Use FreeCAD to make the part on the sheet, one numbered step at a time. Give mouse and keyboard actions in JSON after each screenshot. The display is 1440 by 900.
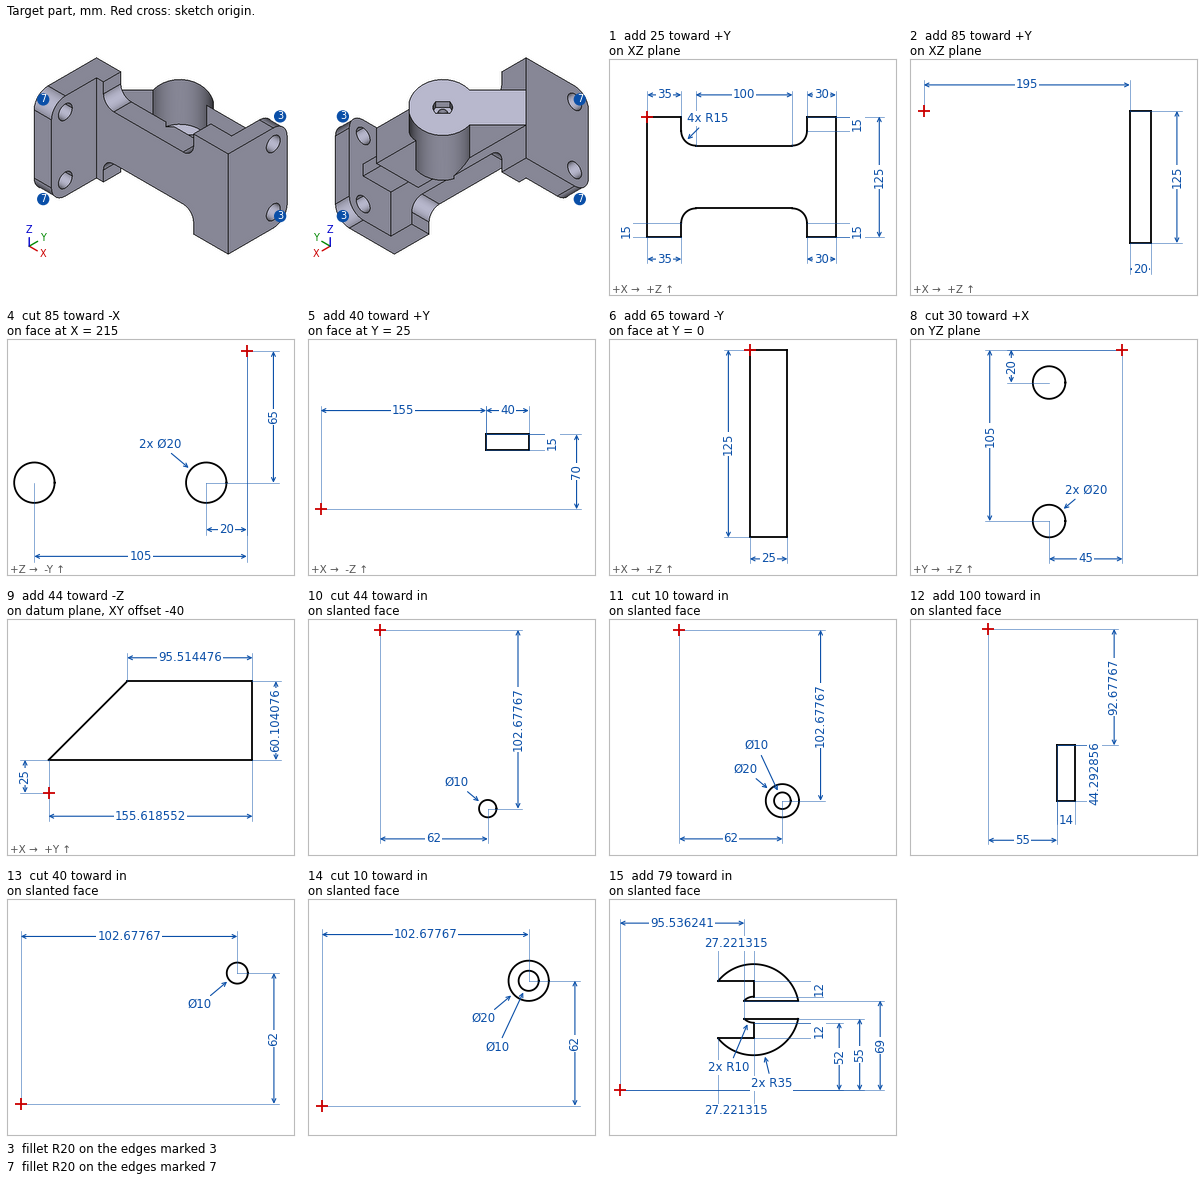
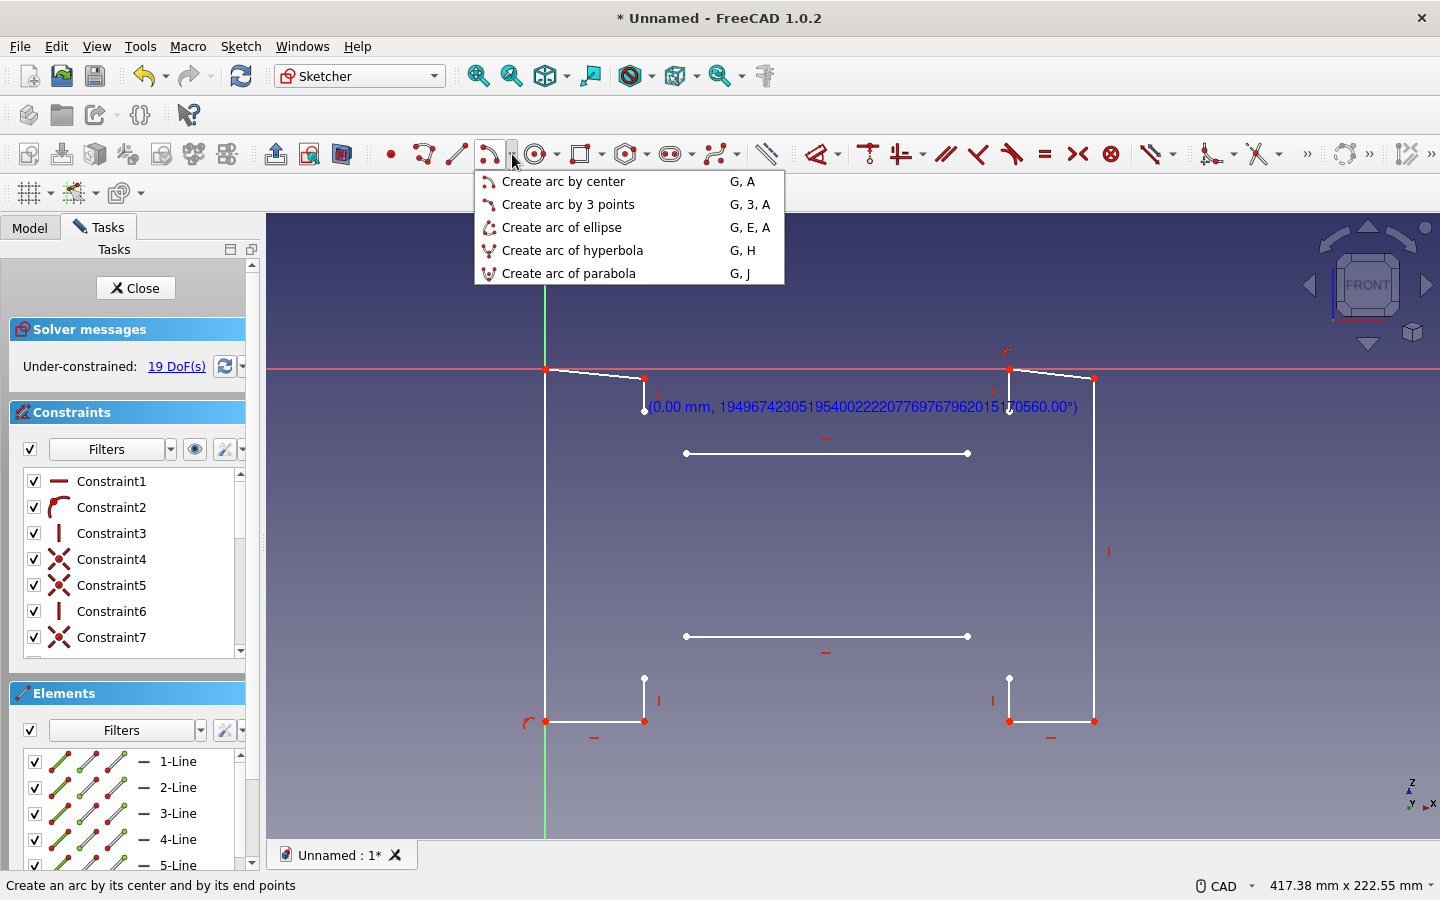
{"action": "left_click", "coordinate": [630, 204]}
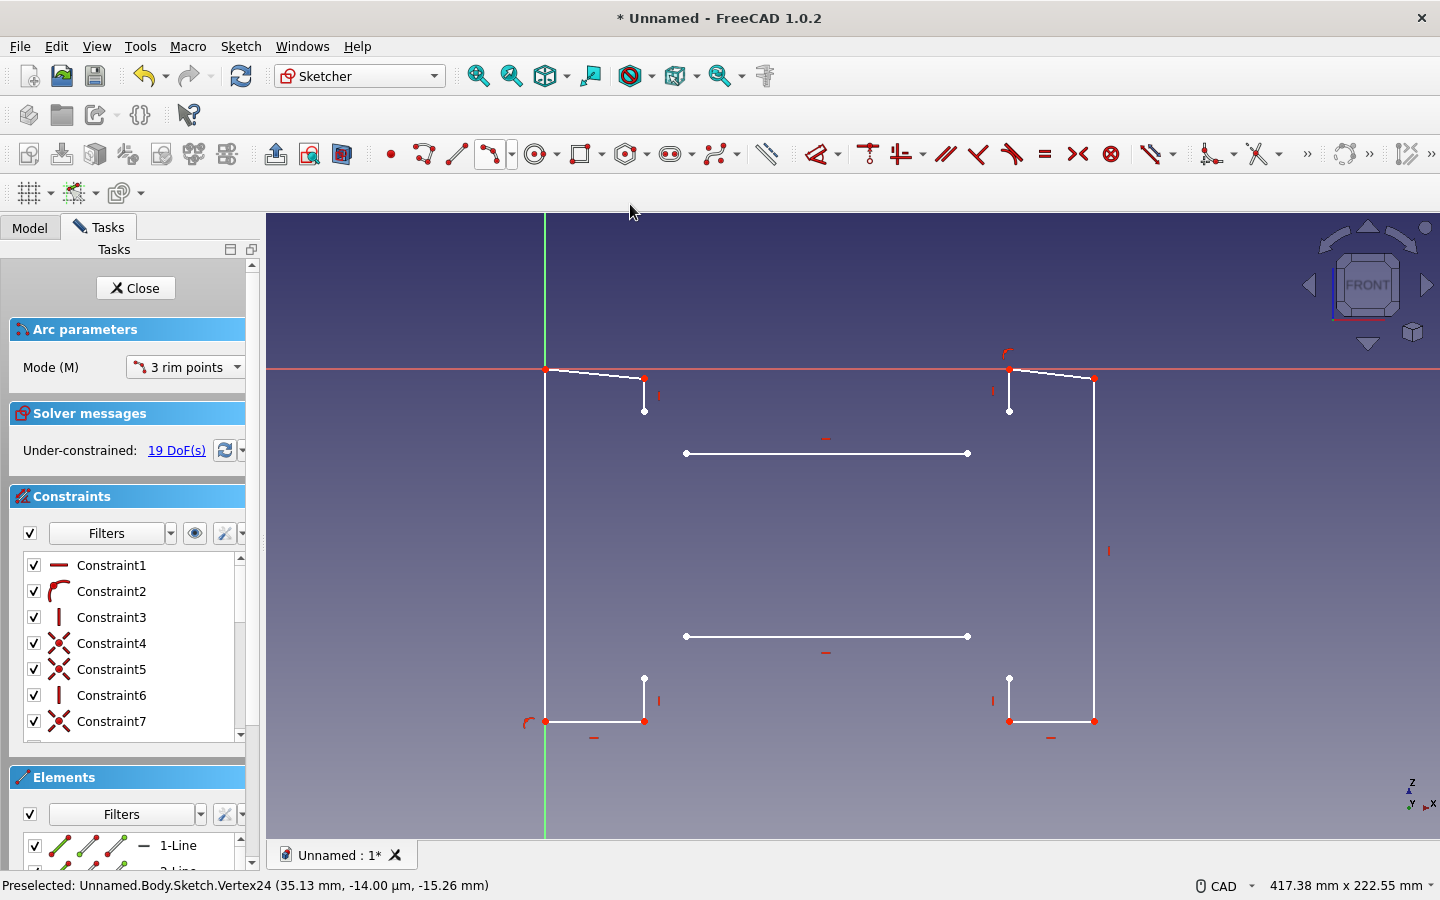
{"action": "left_click", "coordinate": [967, 454]}
{"action": "left_click", "coordinate": [1009, 412]}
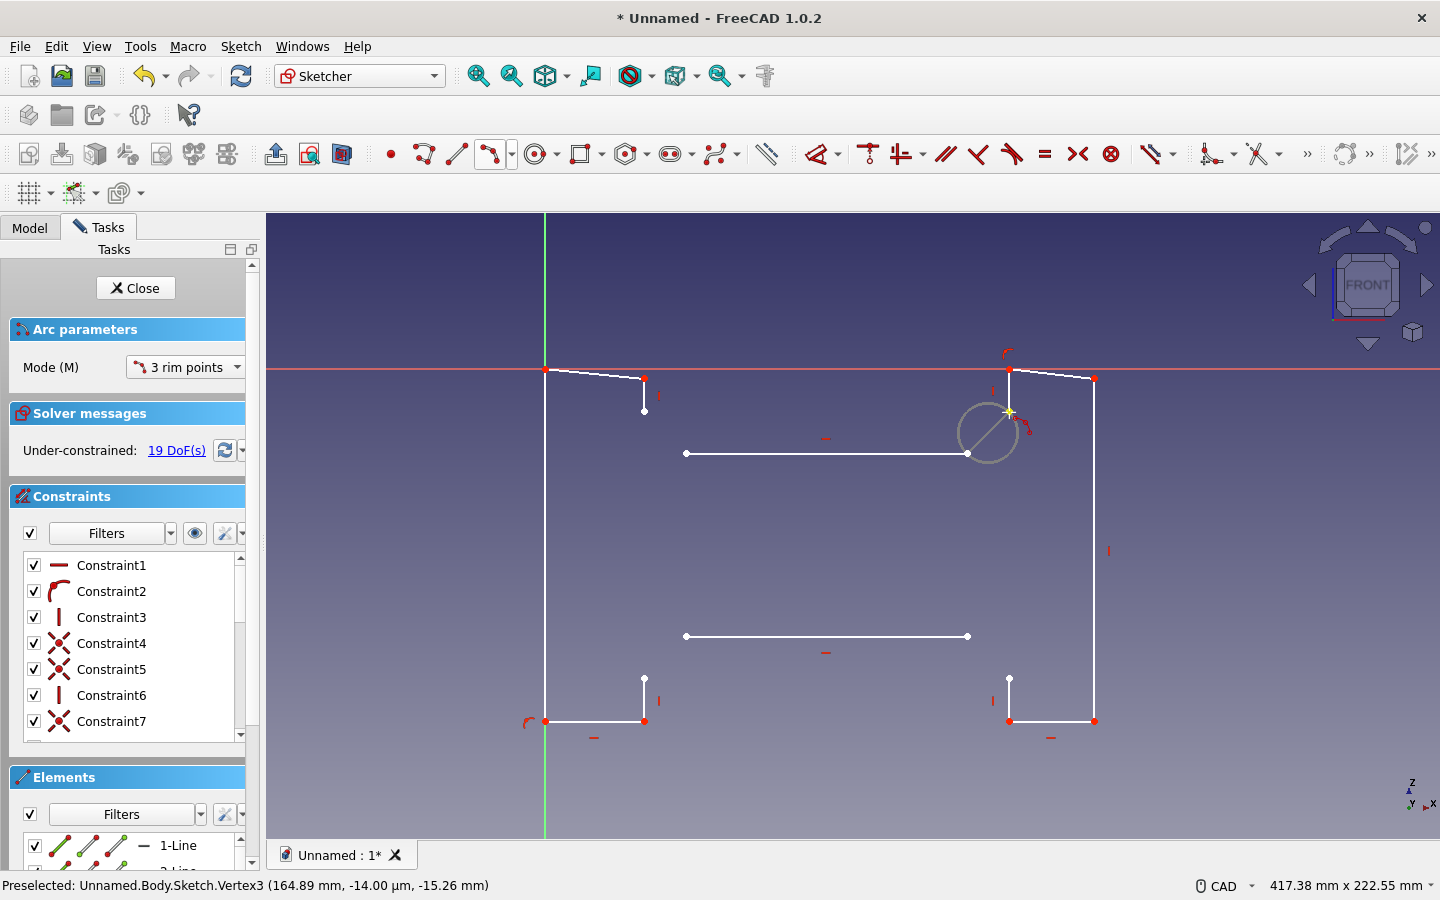
{"action": "scroll", "coordinate": [997, 441], "scroll_direction": "up", "scroll_amount": 2}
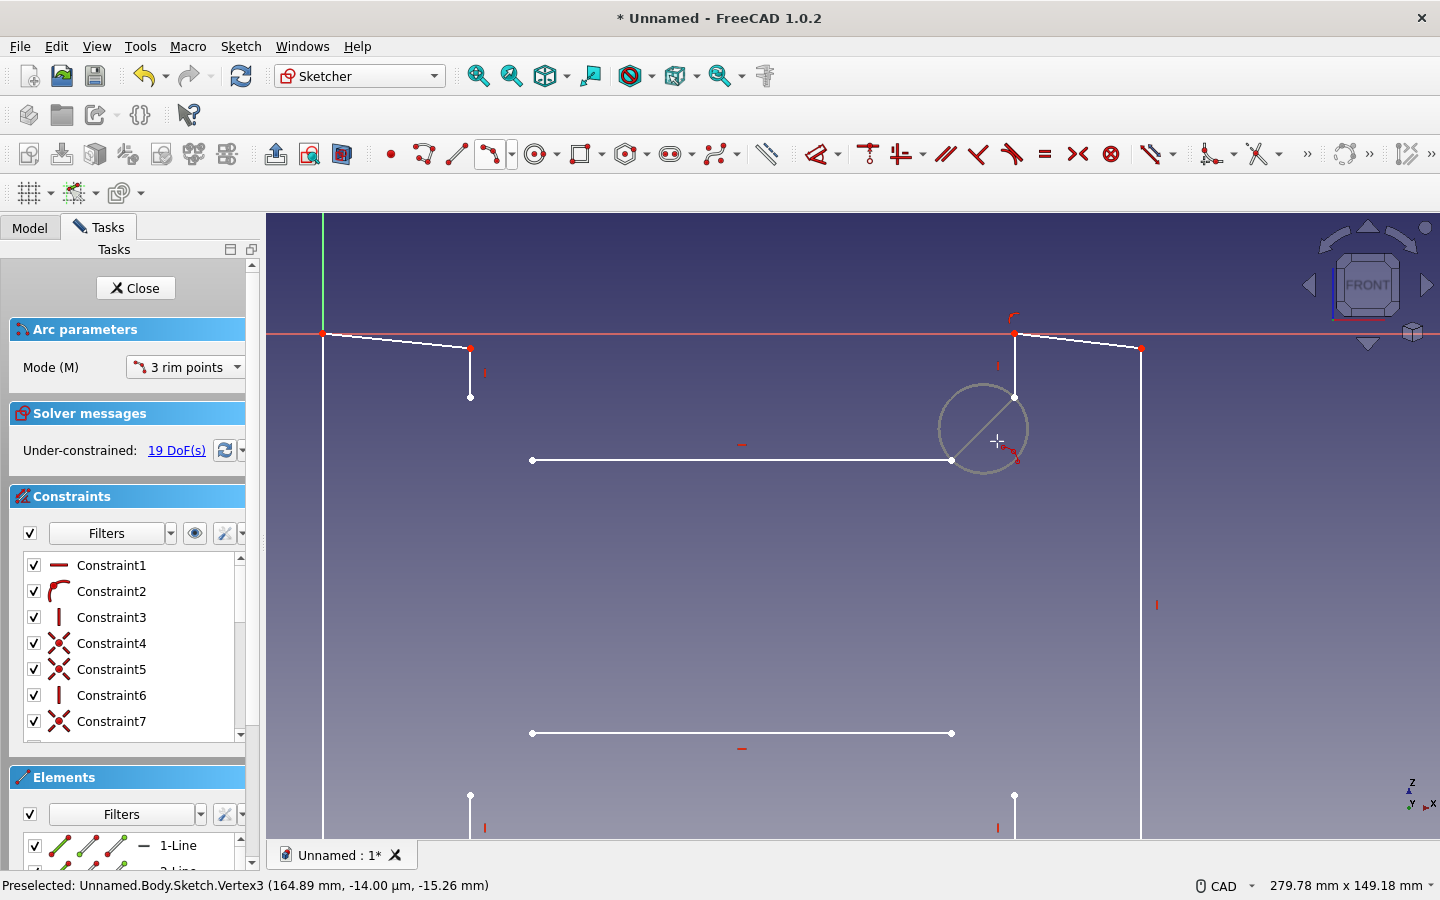
{"action": "left_click", "coordinate": [997, 441]}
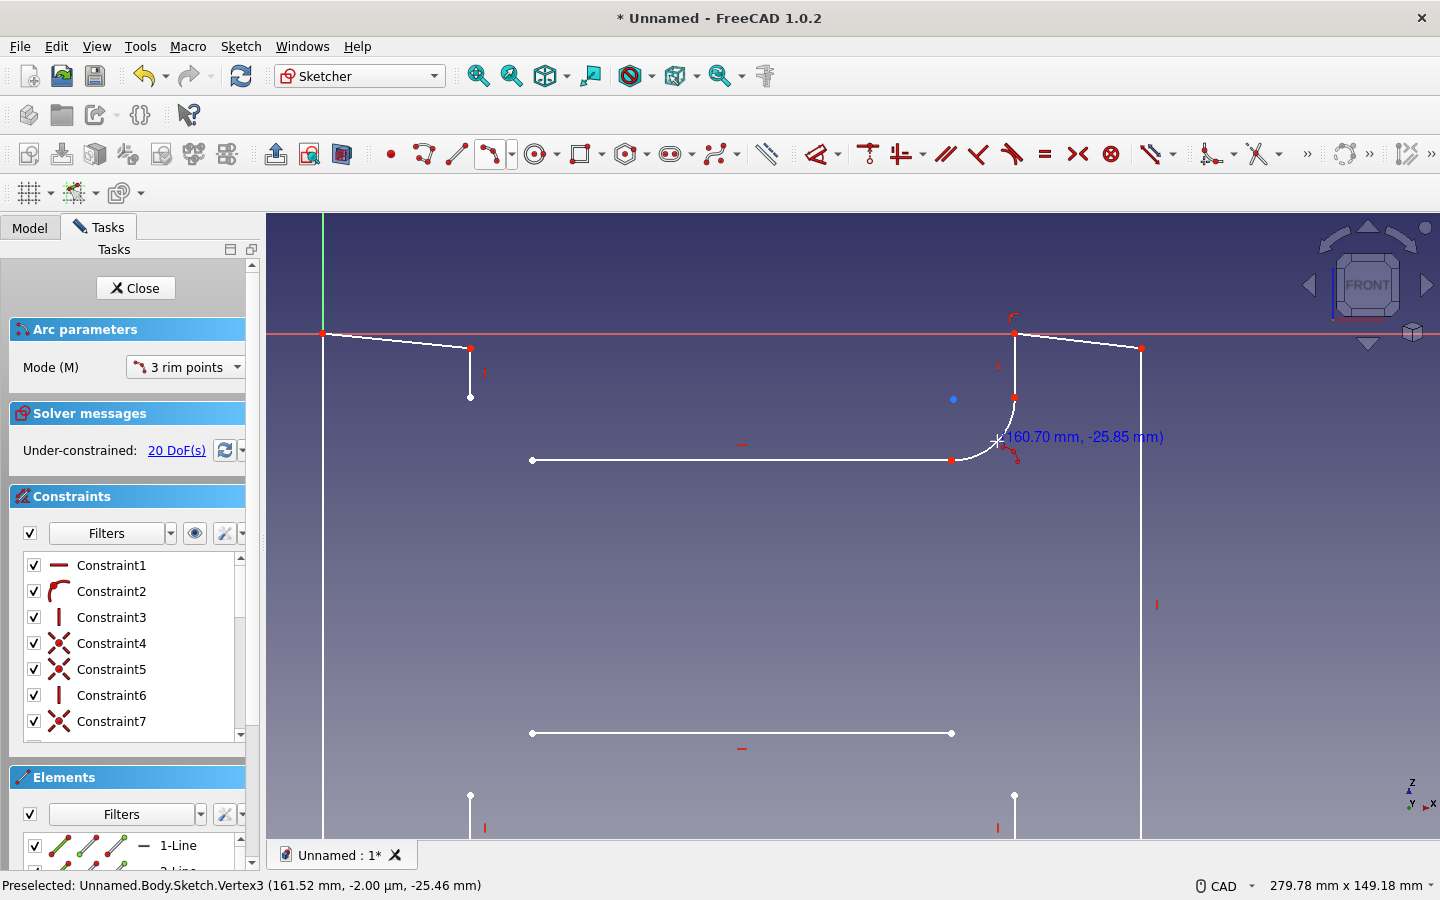
{"action": "left_click", "coordinate": [1015, 796]}
{"action": "left_click", "coordinate": [952, 733]}
{"action": "left_click", "coordinate": [997, 751]}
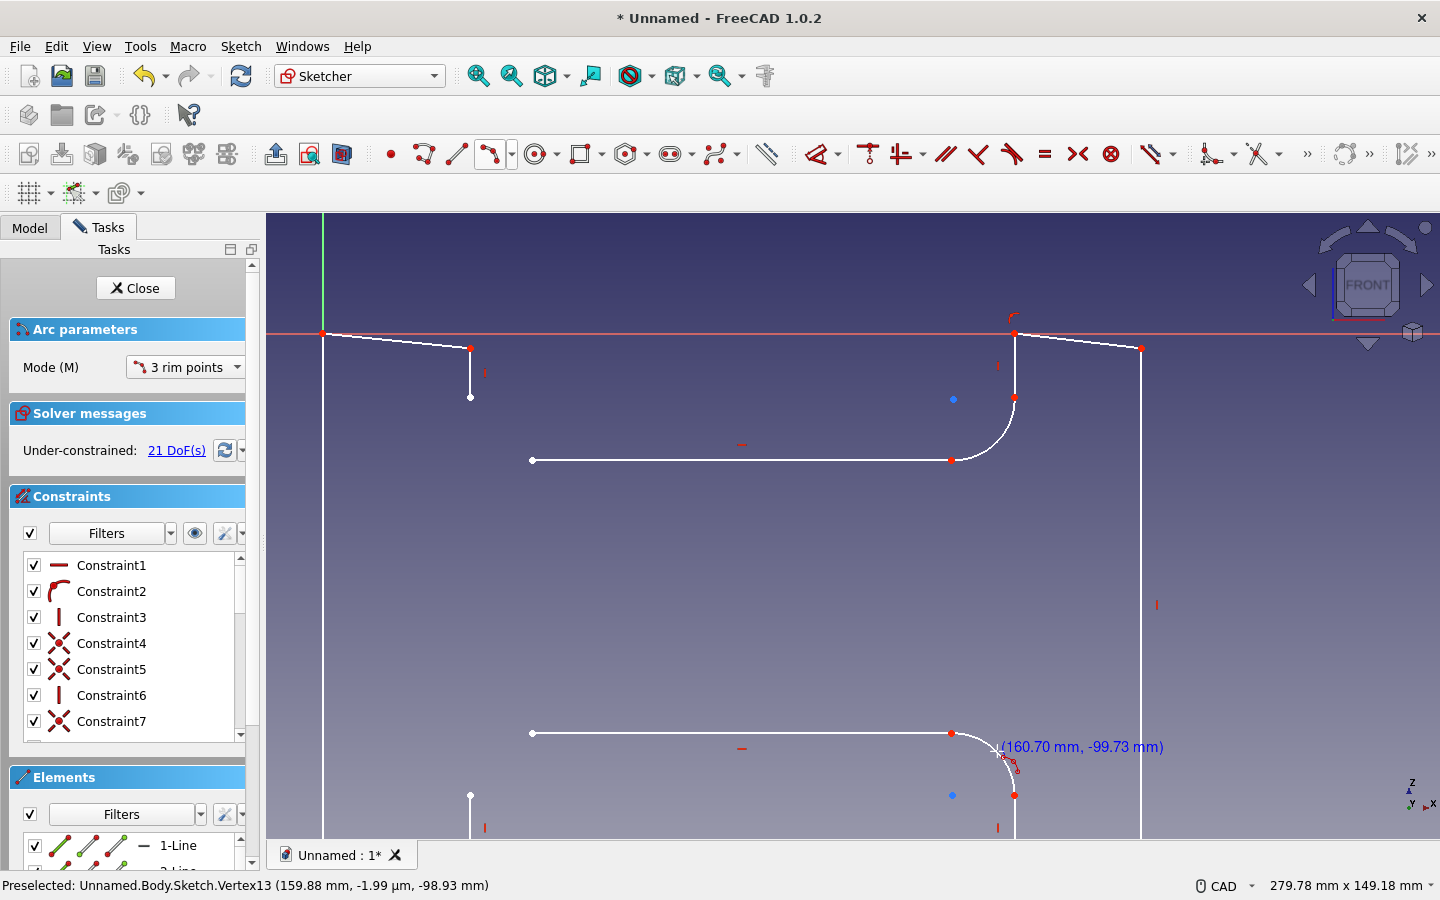
{"action": "left_click", "coordinate": [533, 733]}
{"action": "left_click", "coordinate": [470, 796]}
{"action": "left_click", "coordinate": [488, 751]}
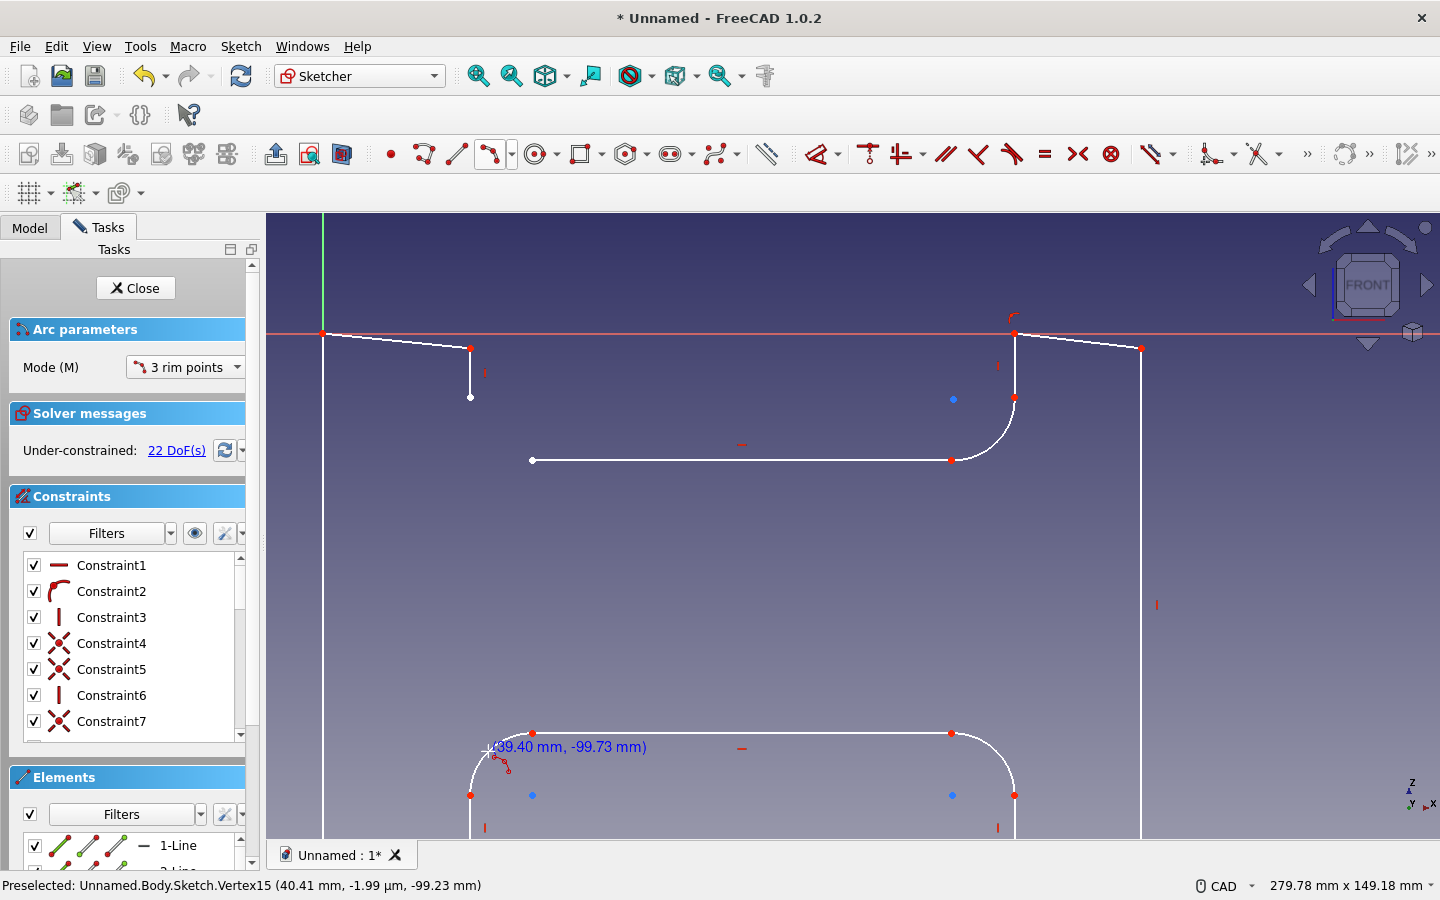
{"action": "left_click", "coordinate": [470, 398]}
{"action": "left_click", "coordinate": [533, 460]}
{"action": "left_click", "coordinate": [488, 441]}
{"action": "key", "text": "Escape"}